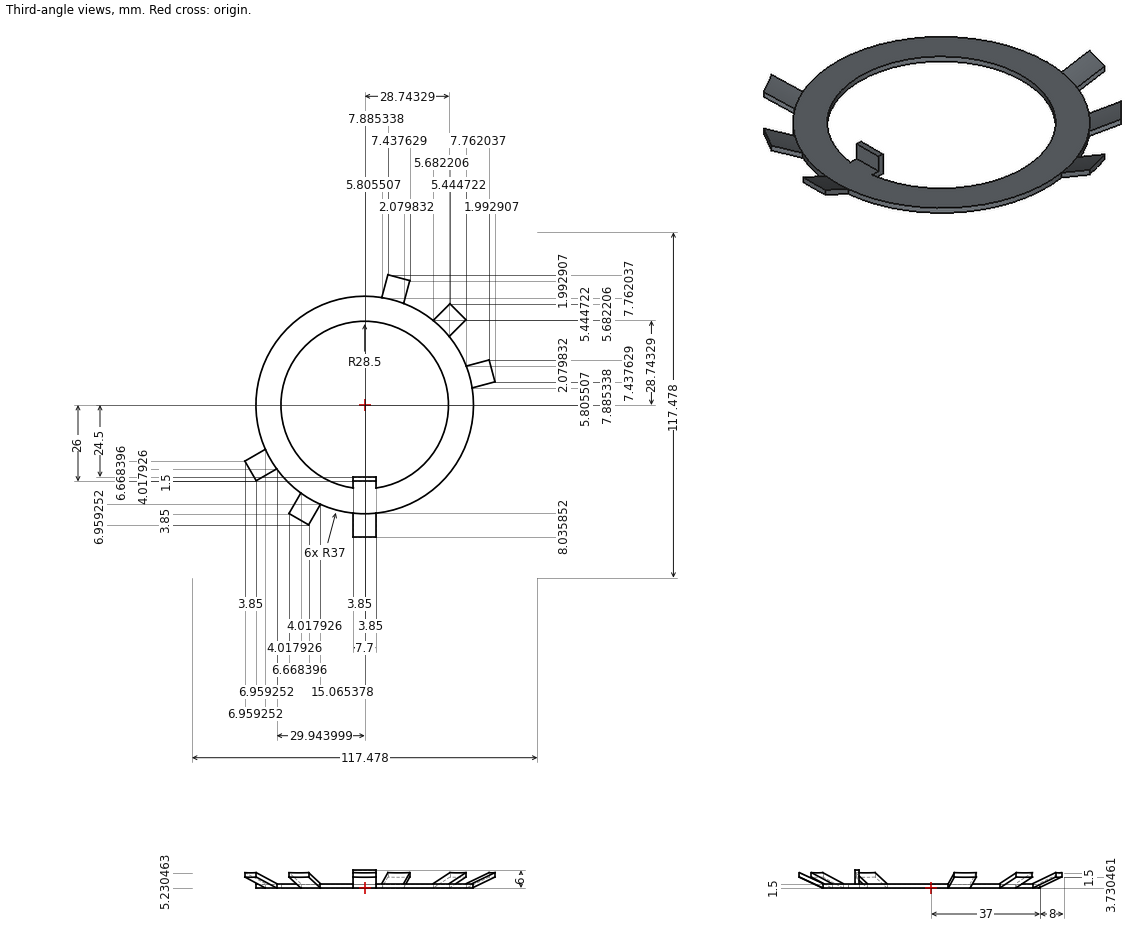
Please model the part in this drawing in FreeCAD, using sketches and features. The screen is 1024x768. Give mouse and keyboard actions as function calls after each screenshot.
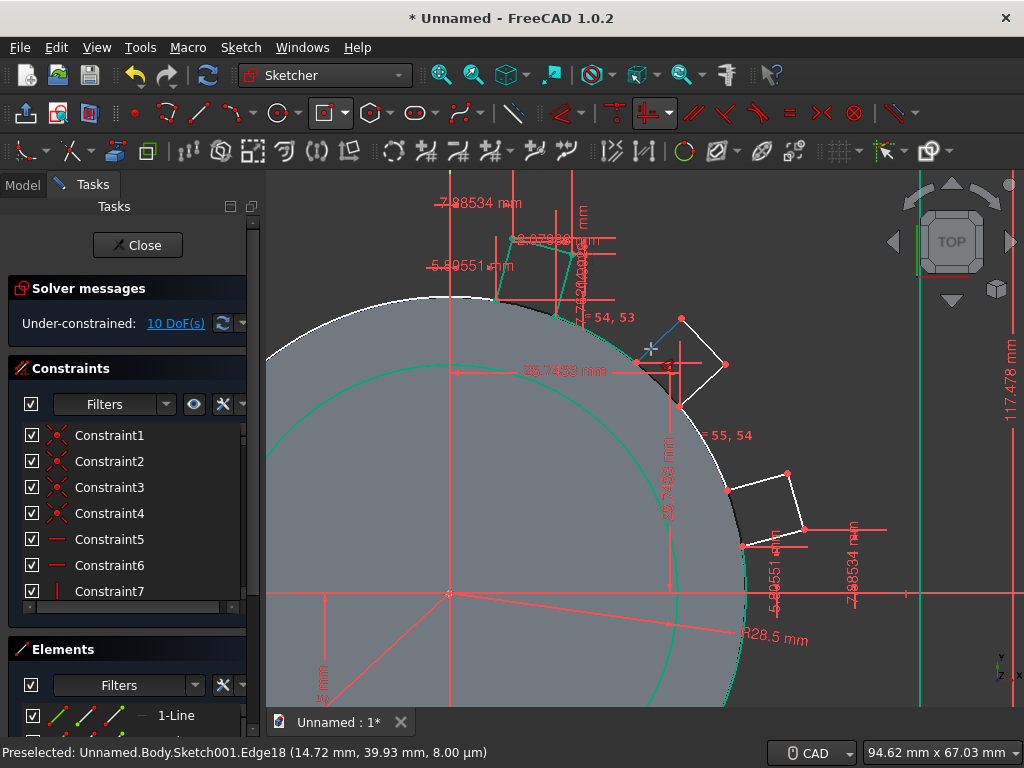
click(650, 350)
click(659, 285)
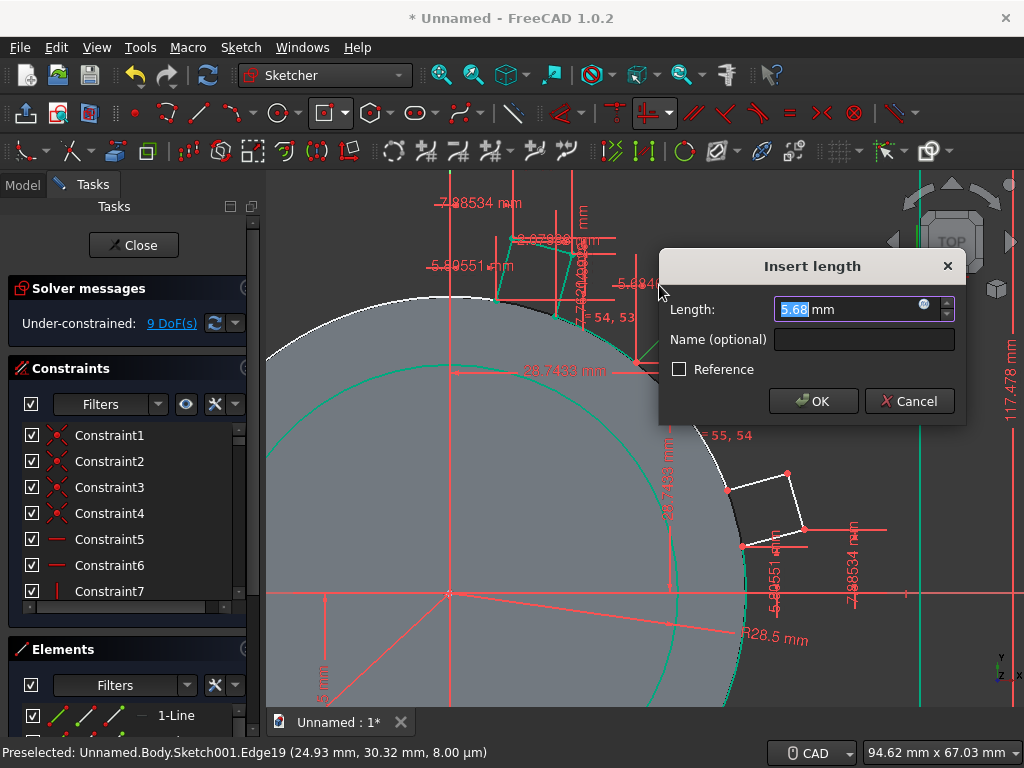
text(5.682206)
key(Return)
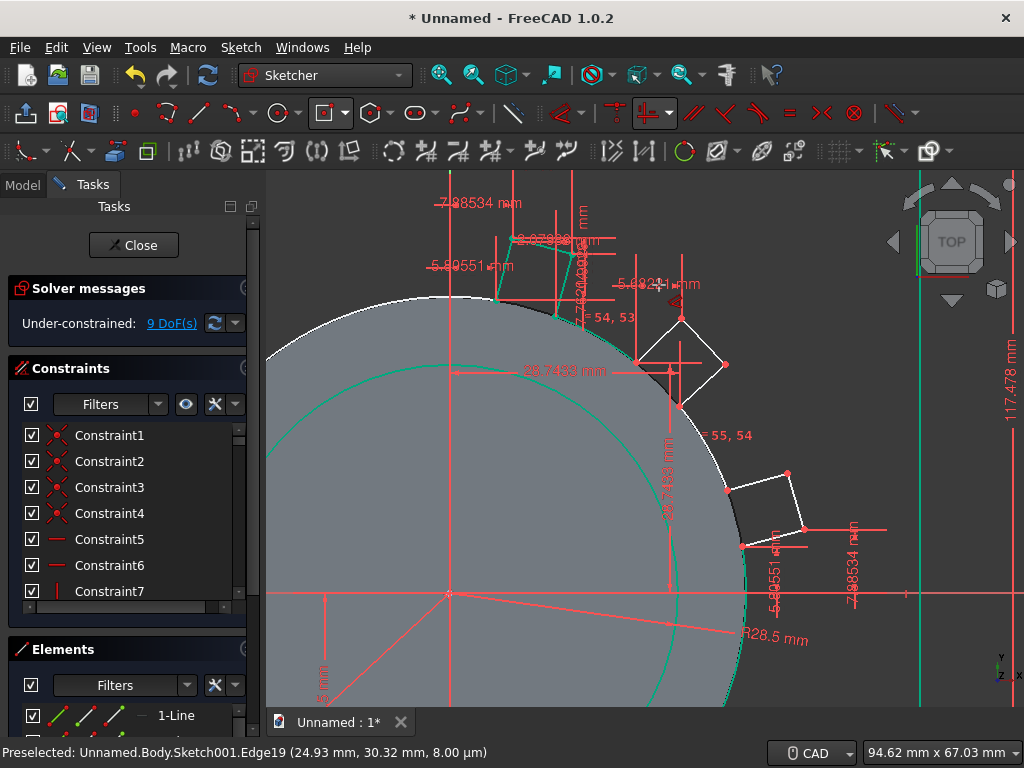
click(650, 350)
click(716, 331)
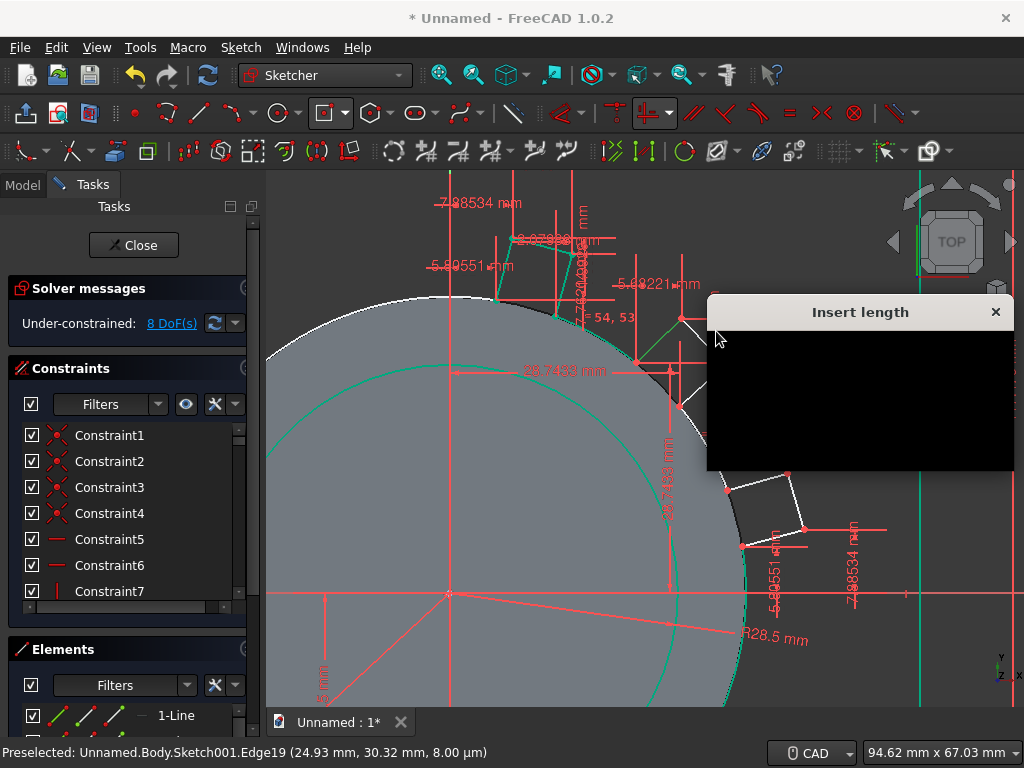
text(5.682206)
key(Return)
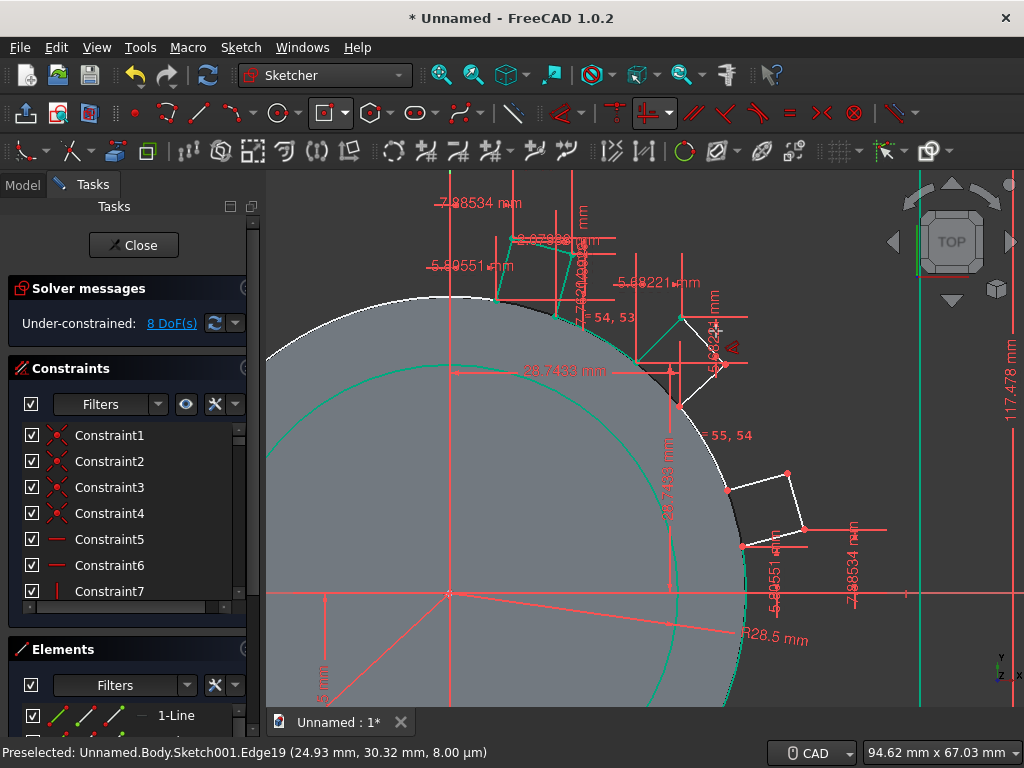
click(695, 332)
click(713, 399)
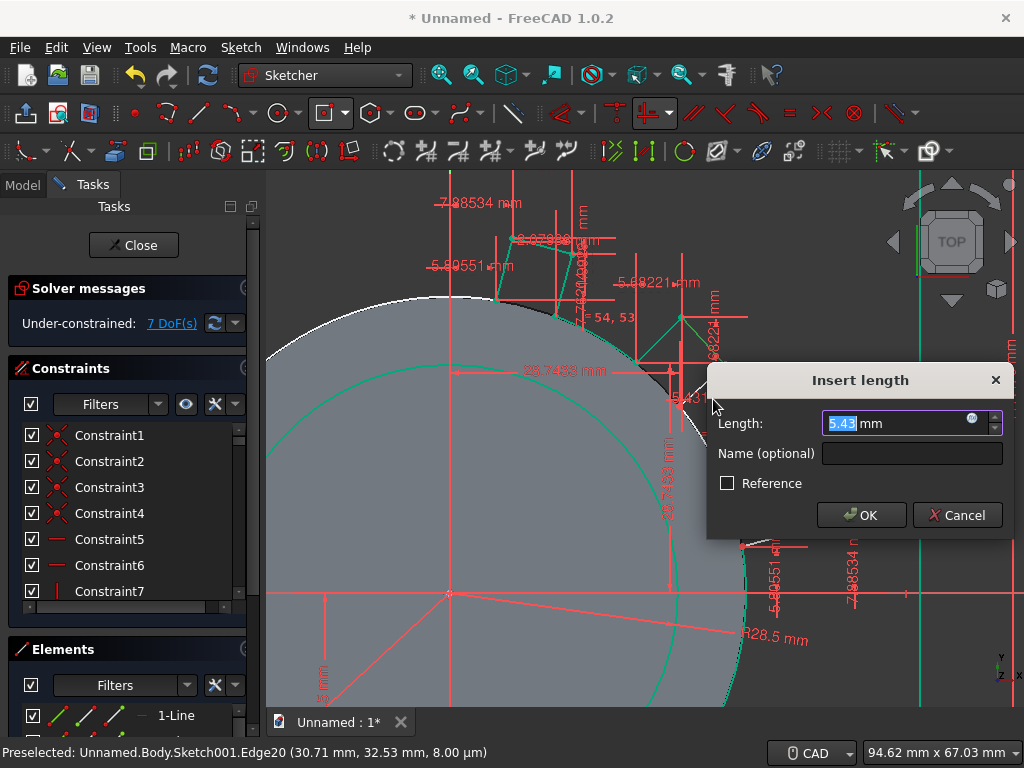
text(5.444722)
key(Return)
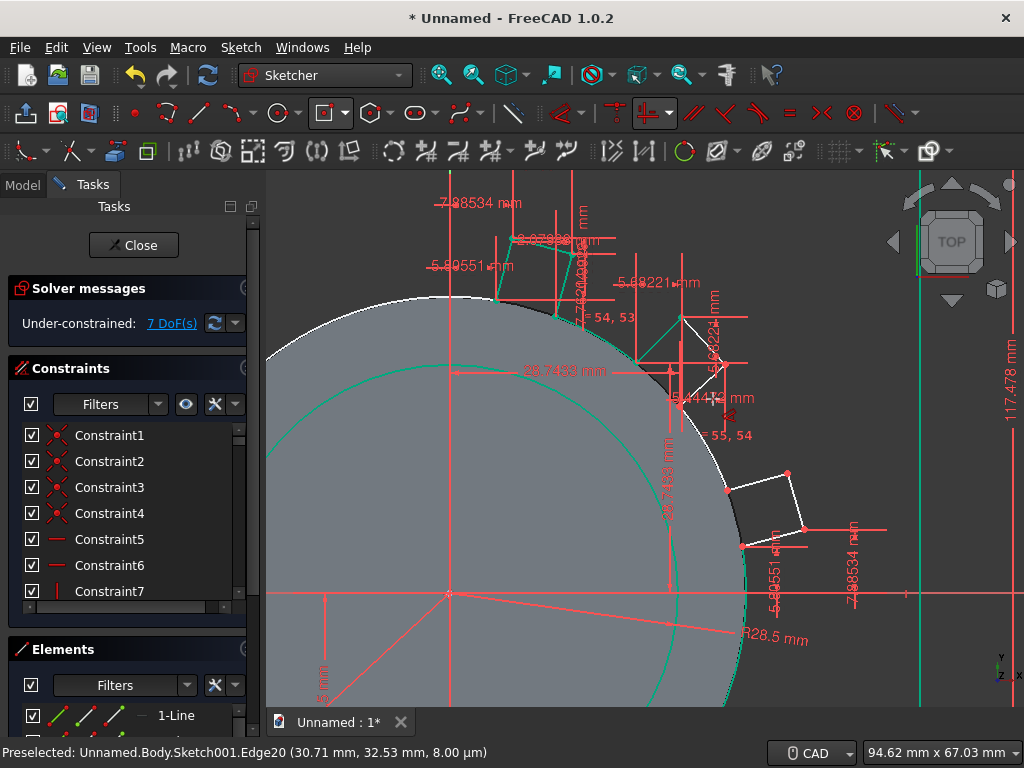
click(695, 332)
click(759, 352)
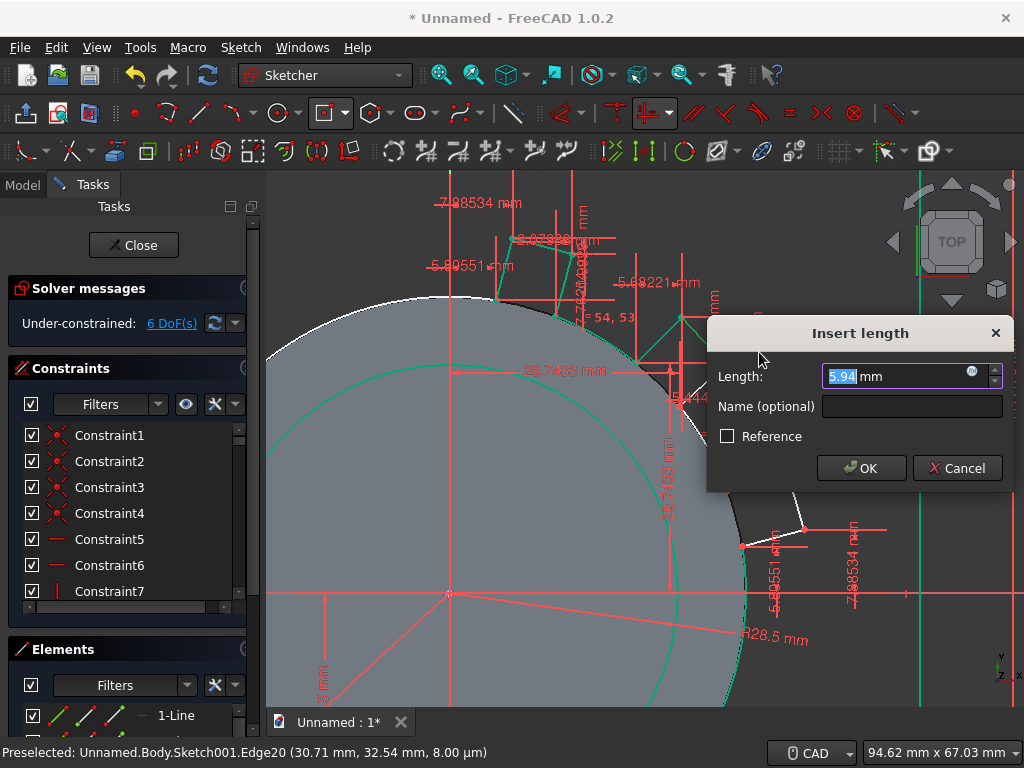
text(5.444722)
key(Return)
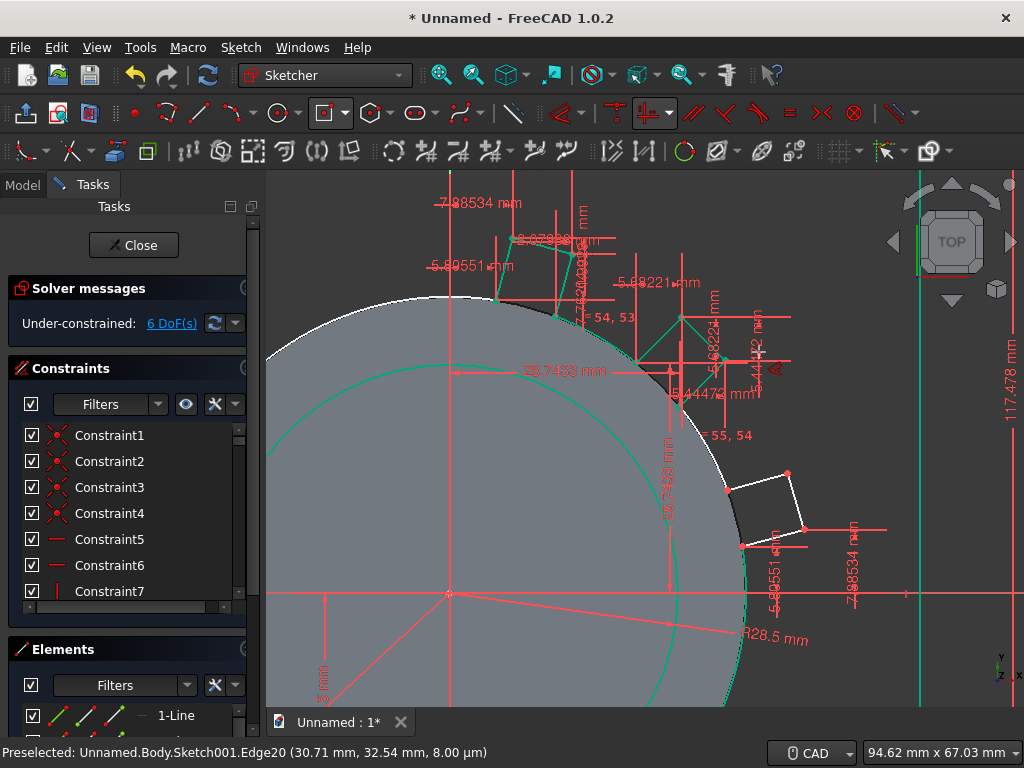
click(746, 485)
click(758, 440)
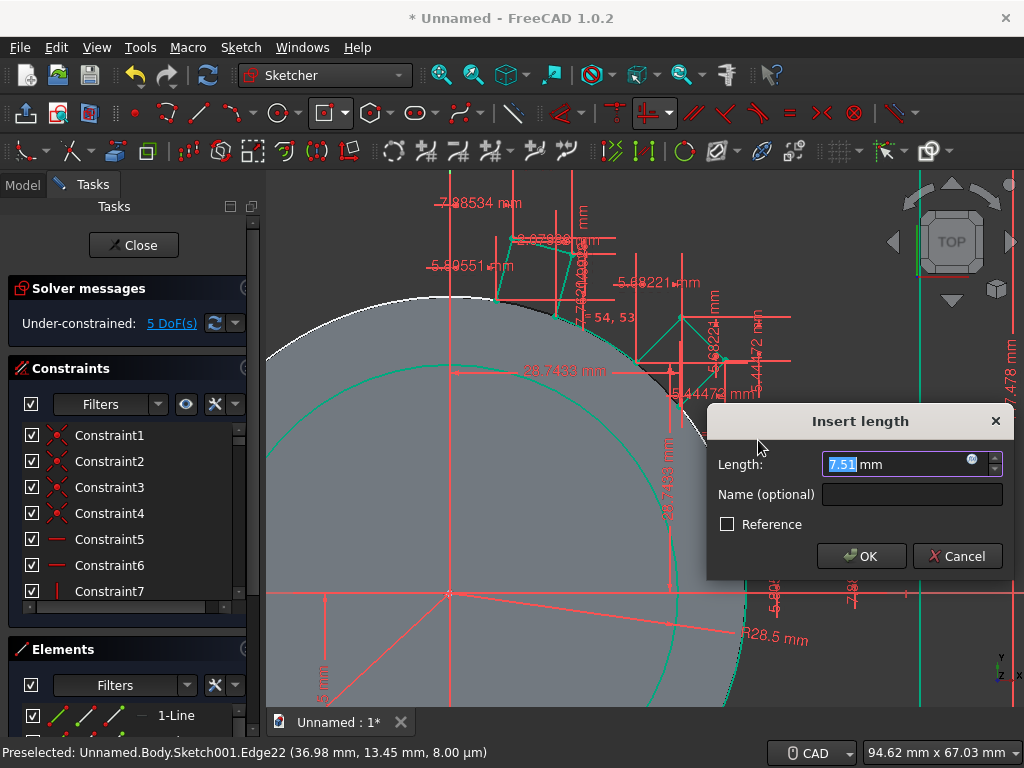
text(7.762037)
key(Return)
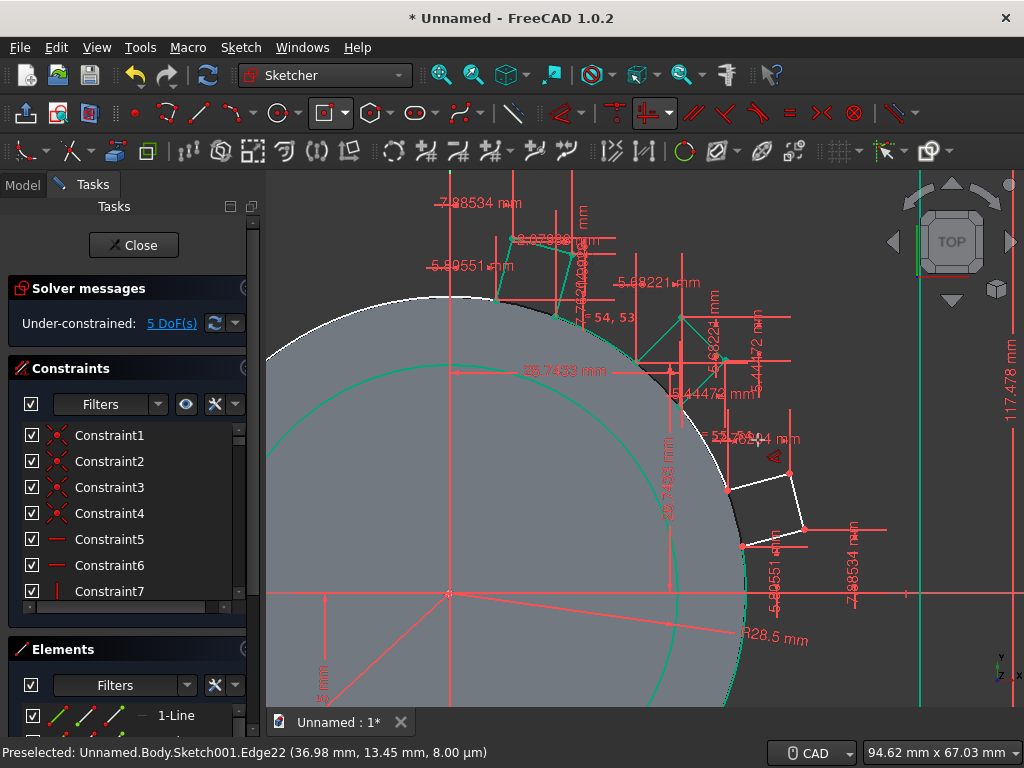
scroll(746, 485, up, 5)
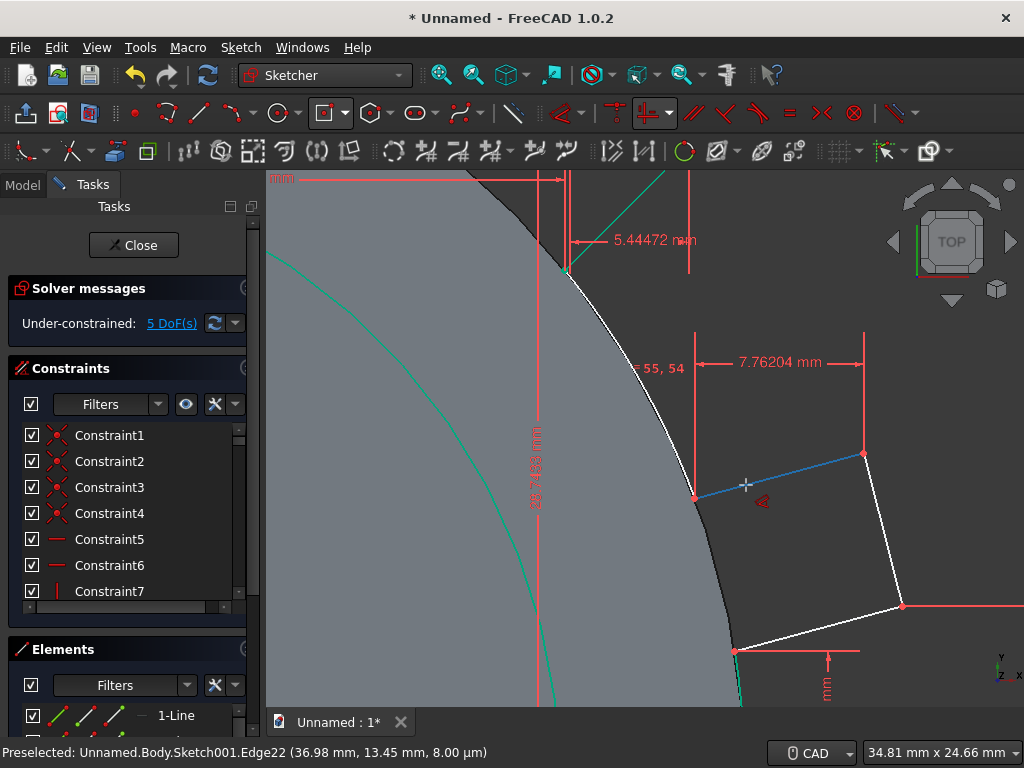
click(746, 485)
click(661, 476)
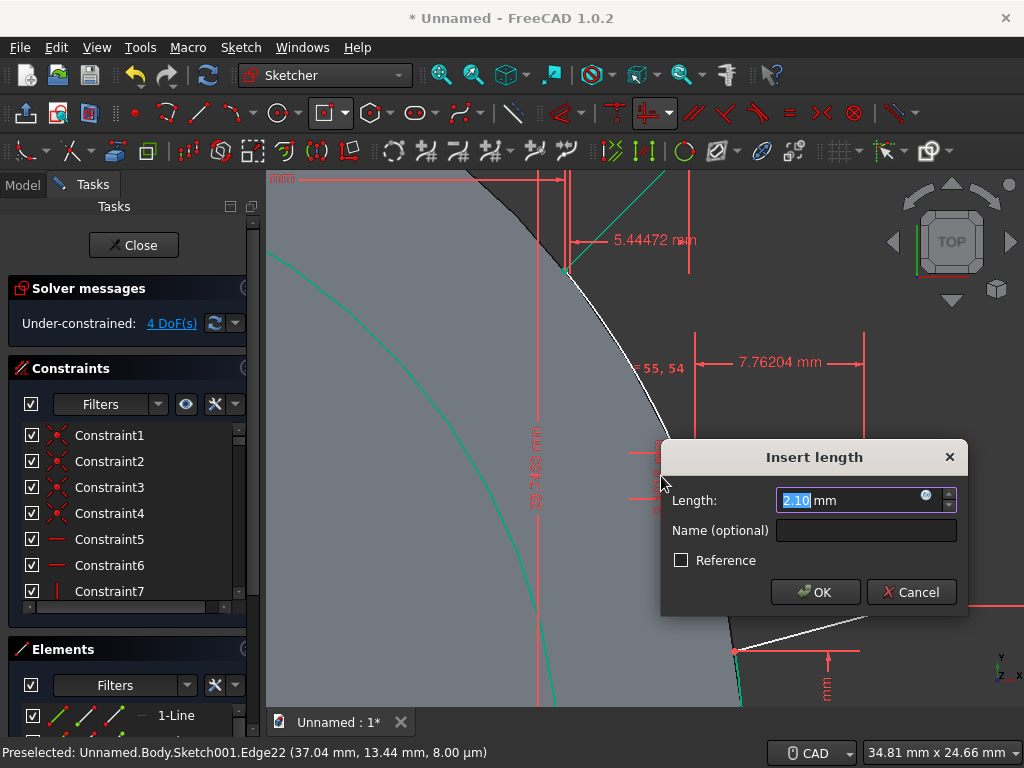
text(2.079832)
key(Return)